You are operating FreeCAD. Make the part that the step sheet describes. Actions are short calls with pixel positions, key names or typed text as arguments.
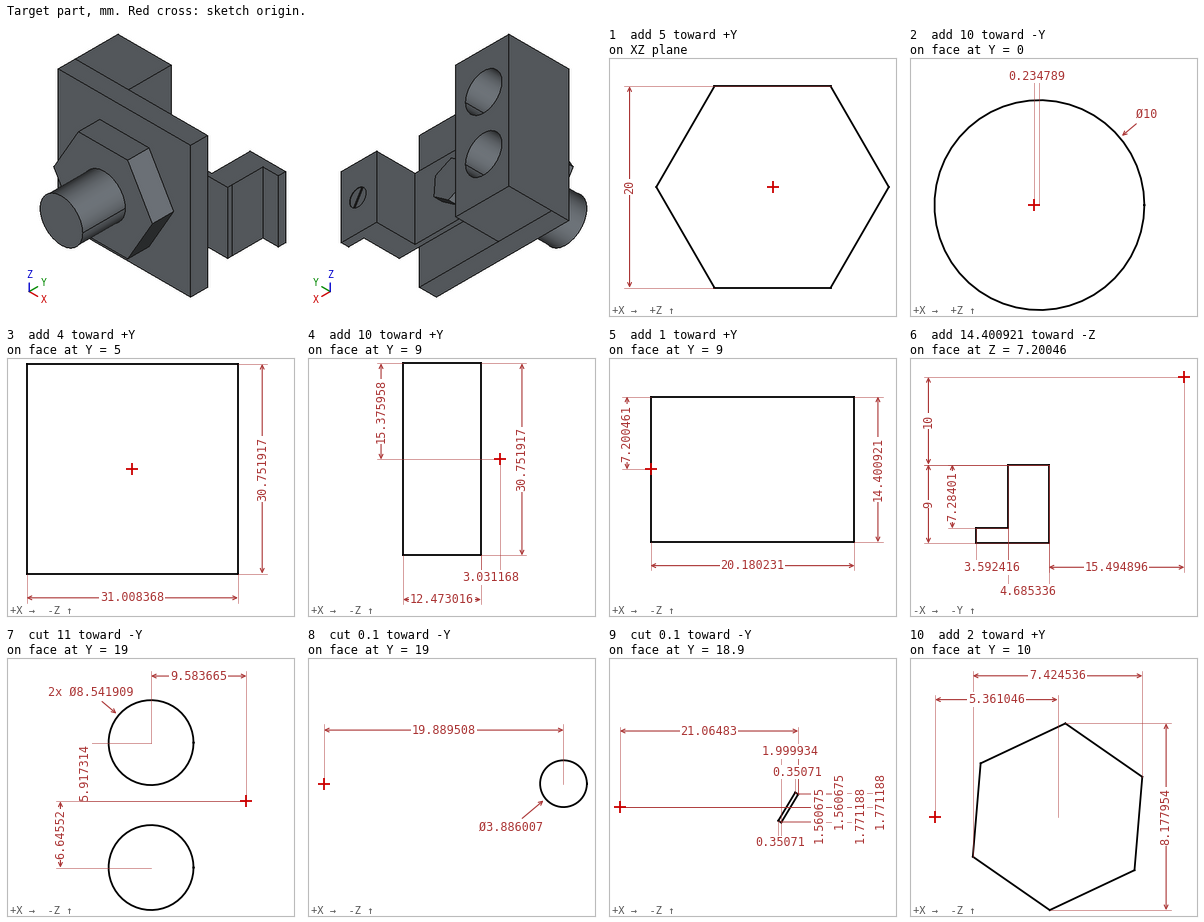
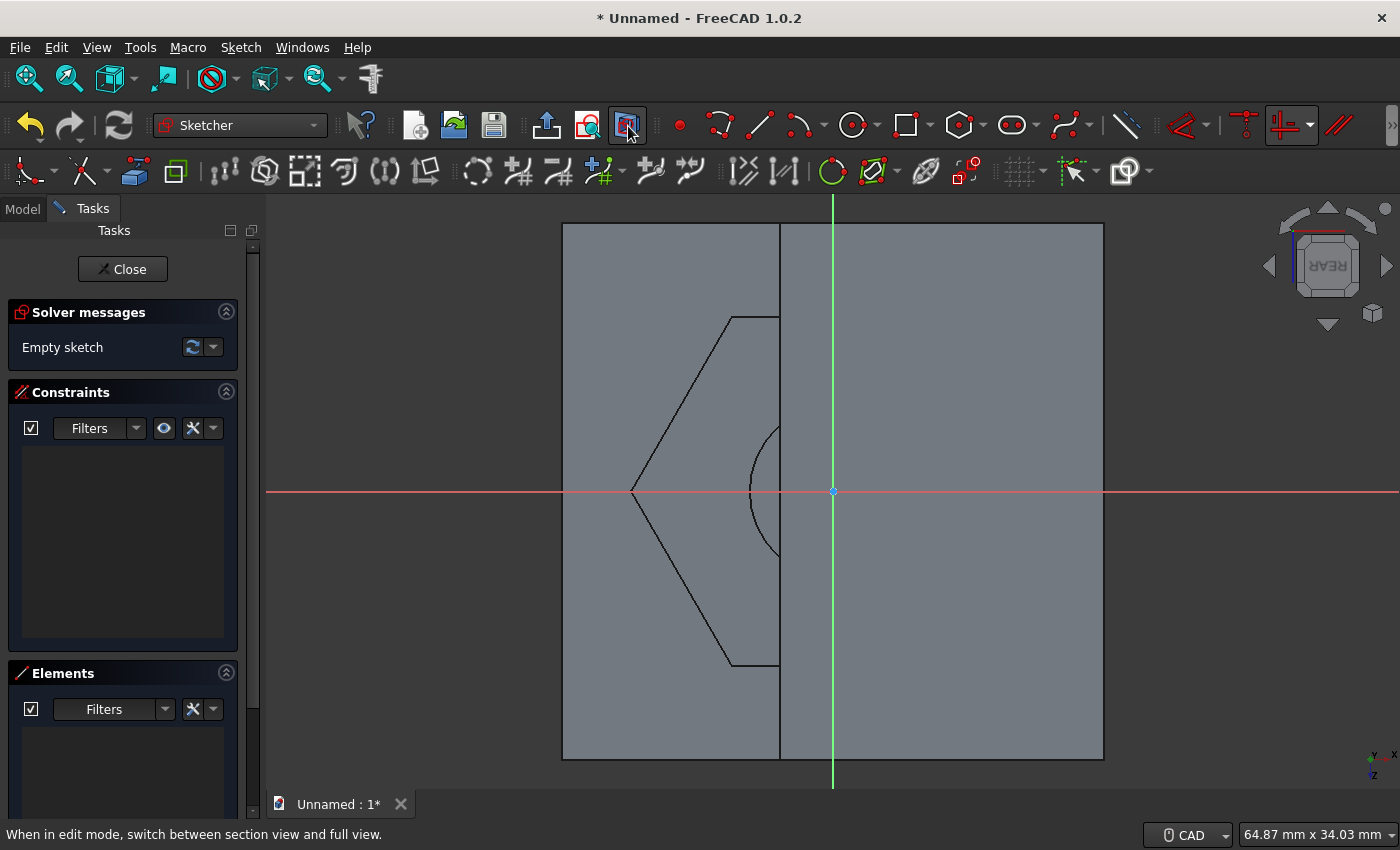
scroll(1235, 491, up, 2)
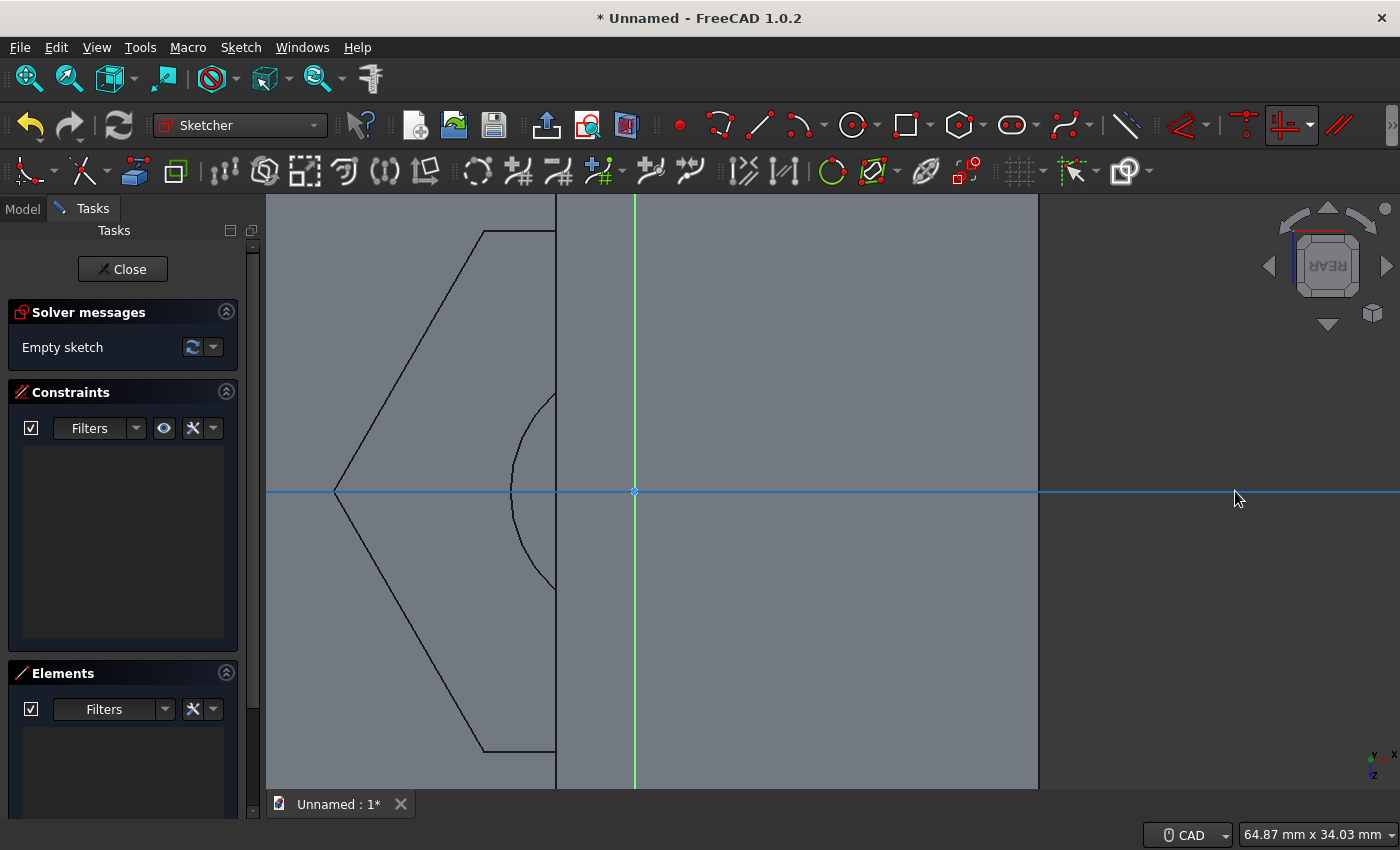
click(906, 126)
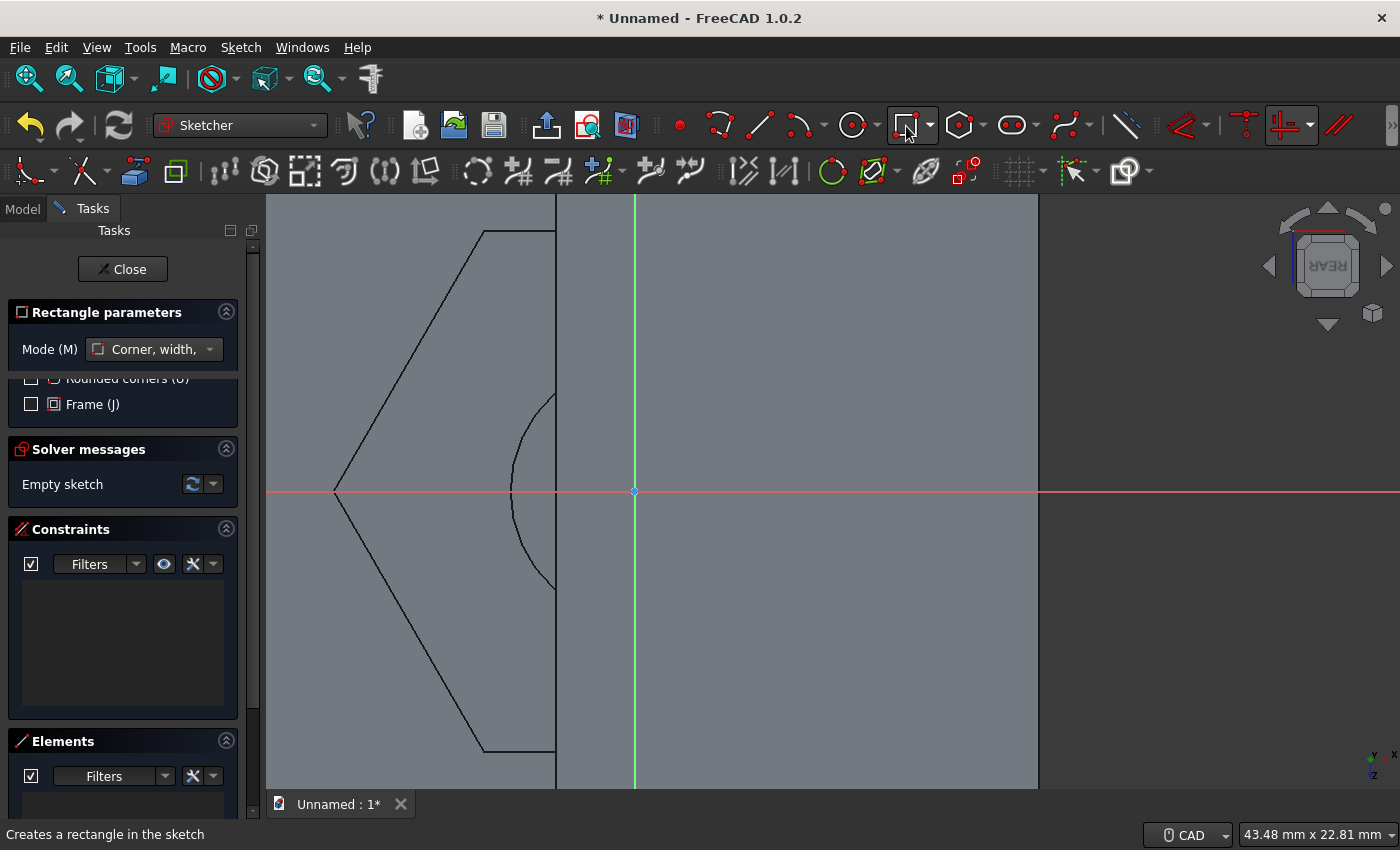
click(635, 304)
move(1161, 679)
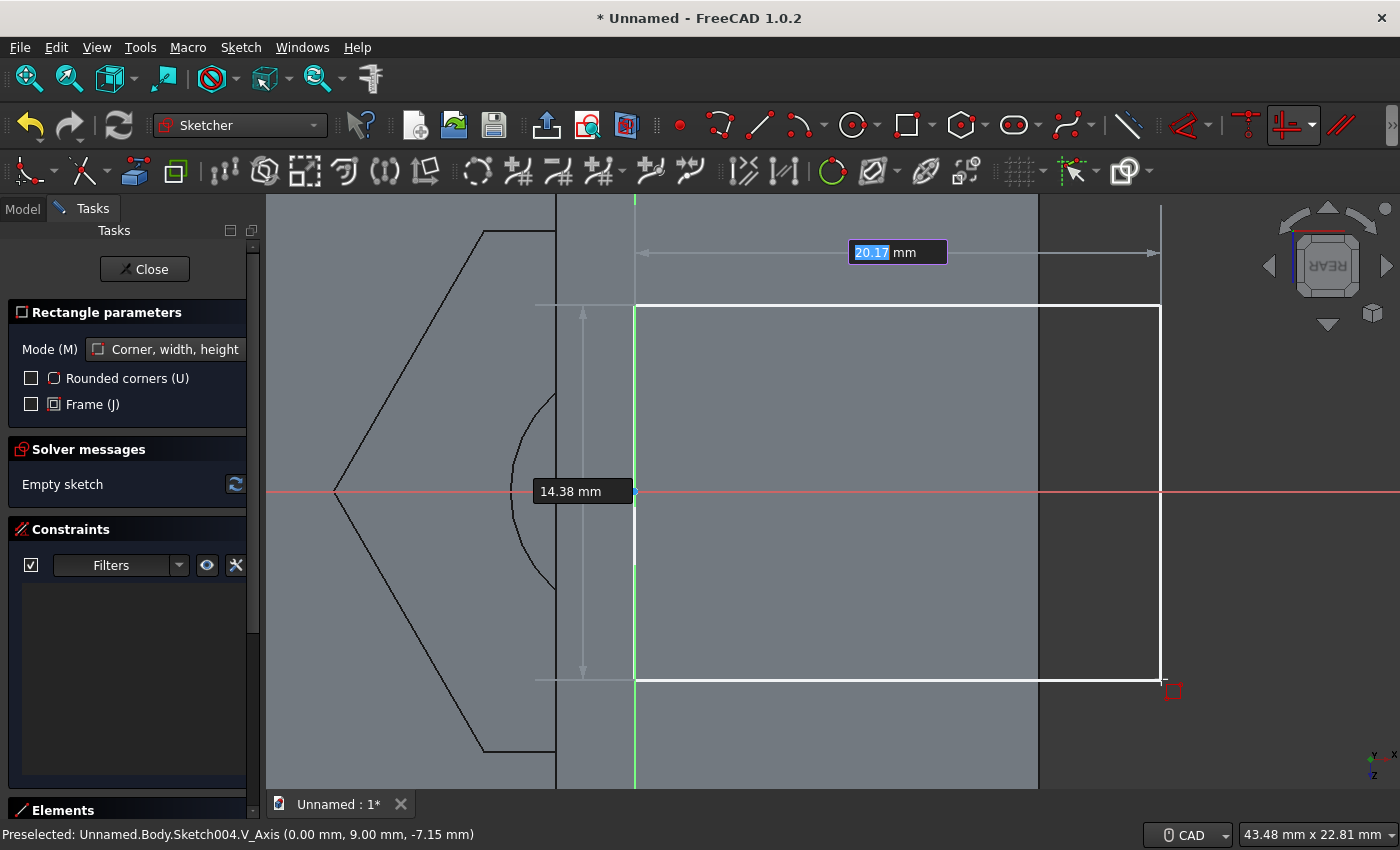
text(20.180231)
key(Tab)
text(14.400921)
key(Return)
key(Escape)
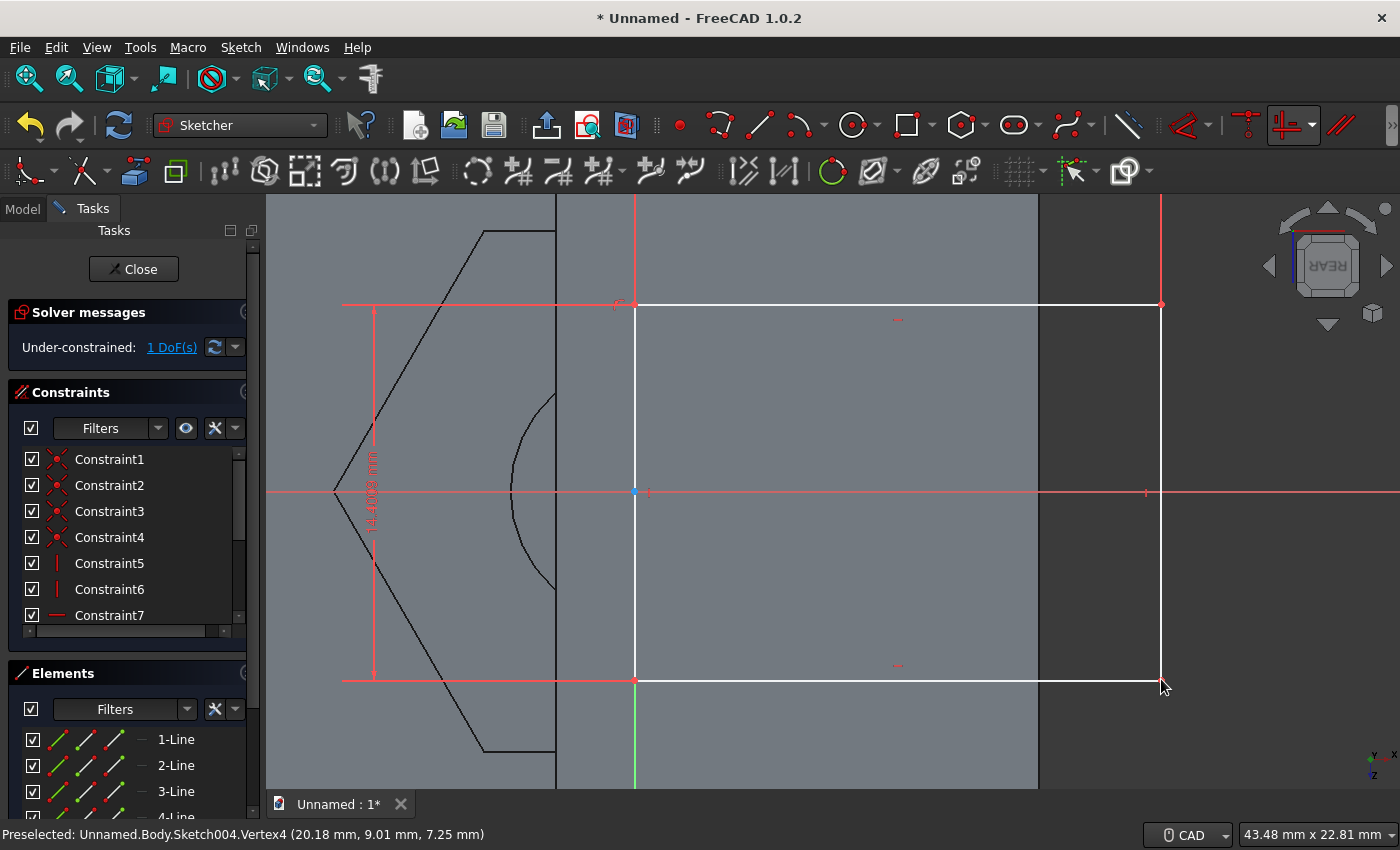
click(1184, 126)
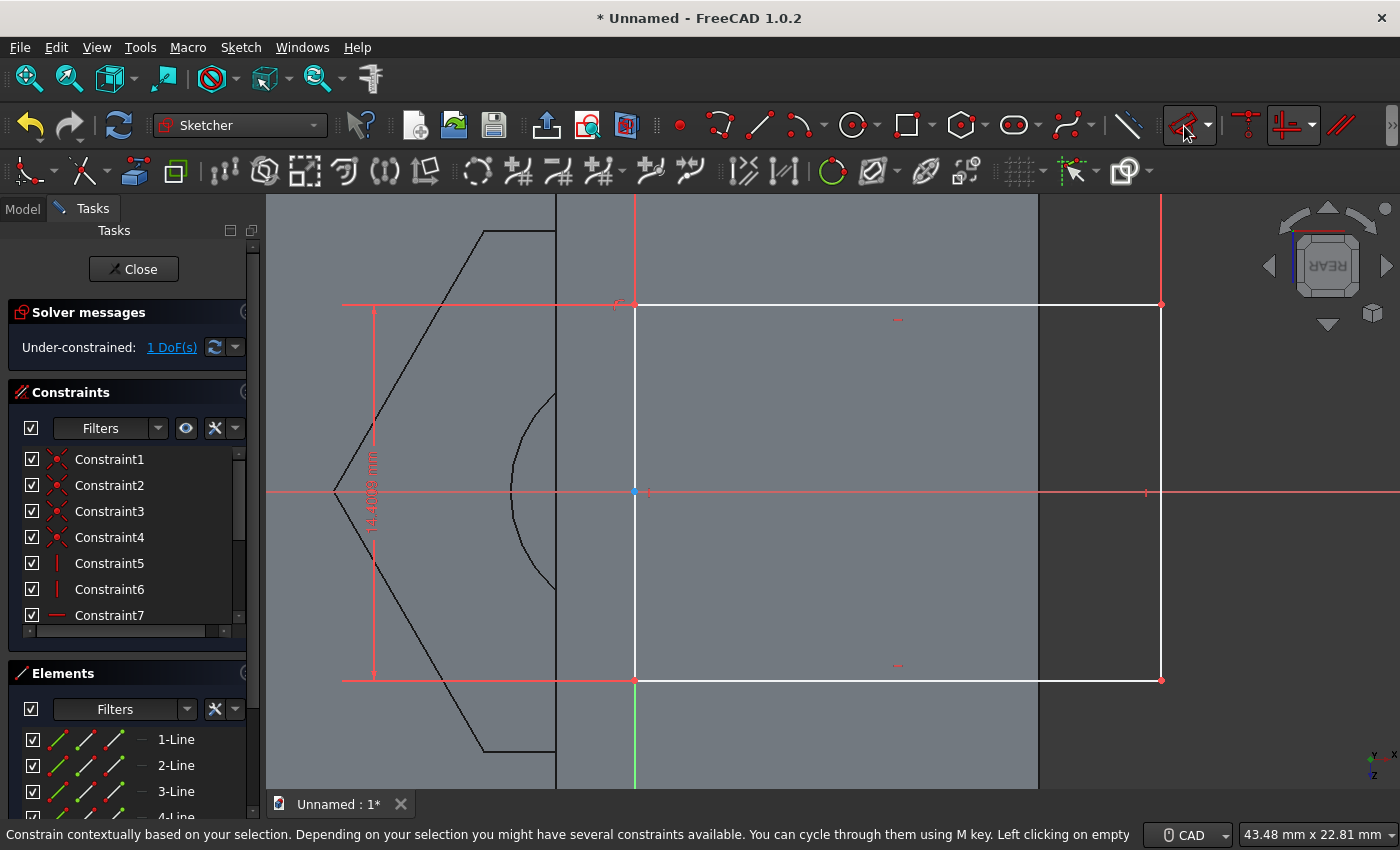
click(635, 305)
click(601, 398)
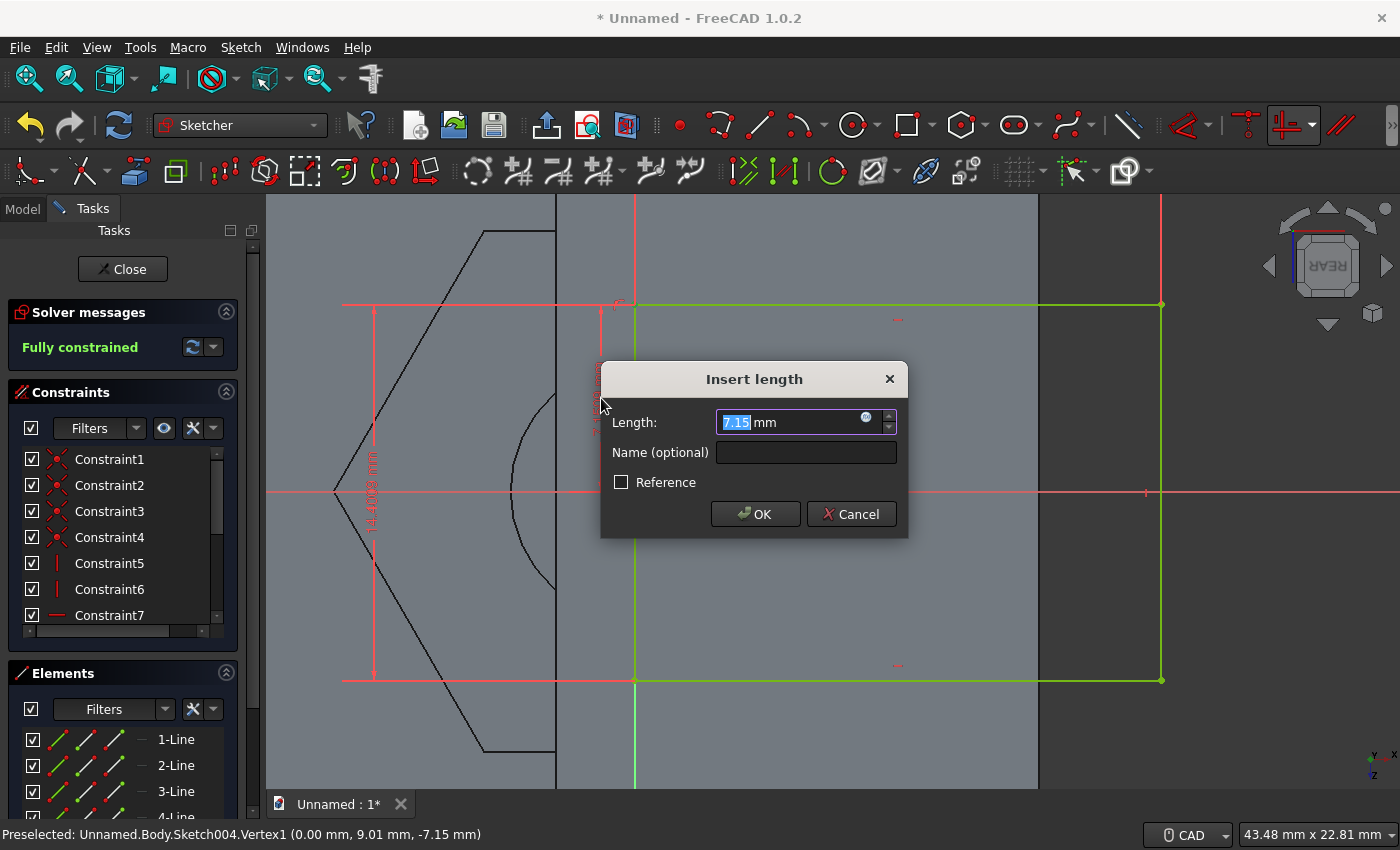
text(7.200461)
key(Return)
key(Escape)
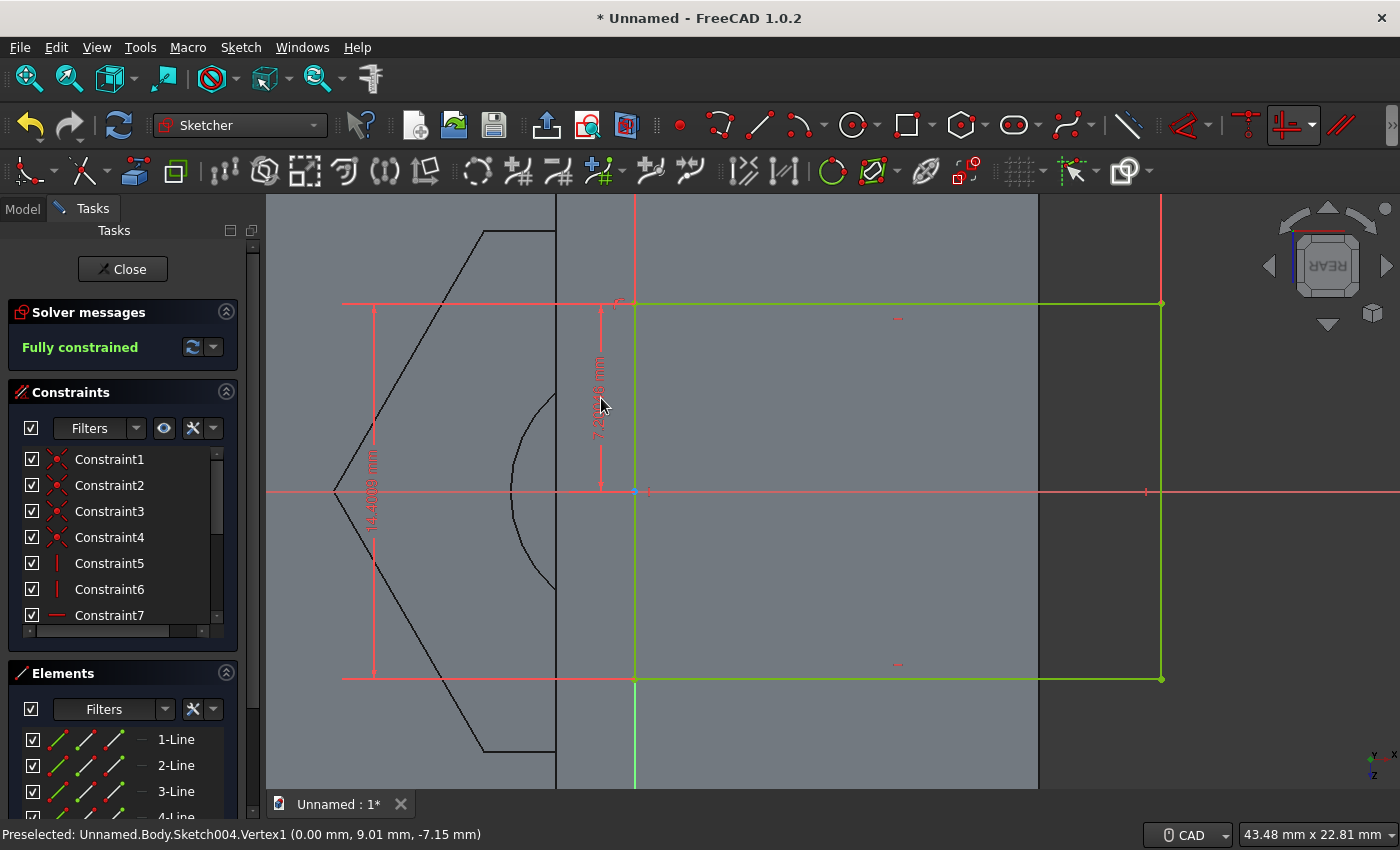
click(123, 269)